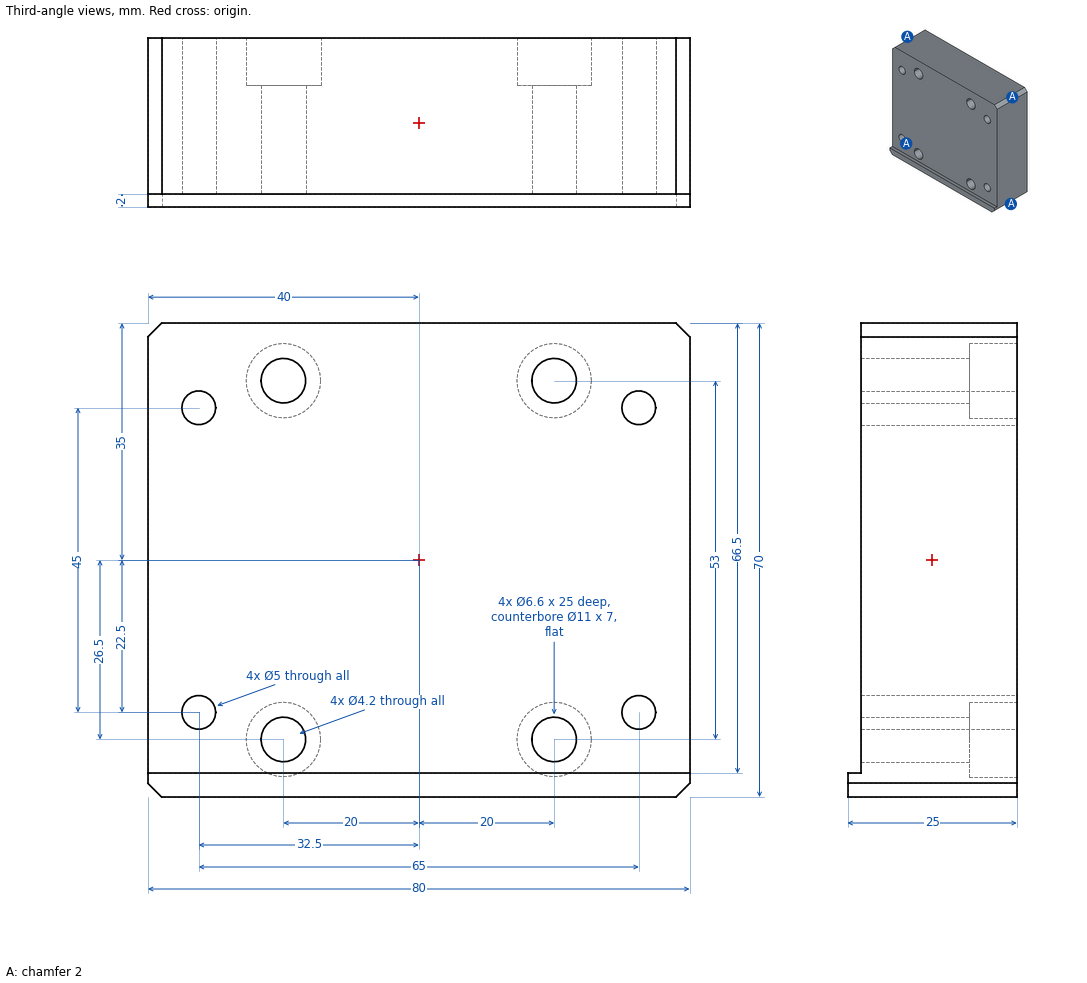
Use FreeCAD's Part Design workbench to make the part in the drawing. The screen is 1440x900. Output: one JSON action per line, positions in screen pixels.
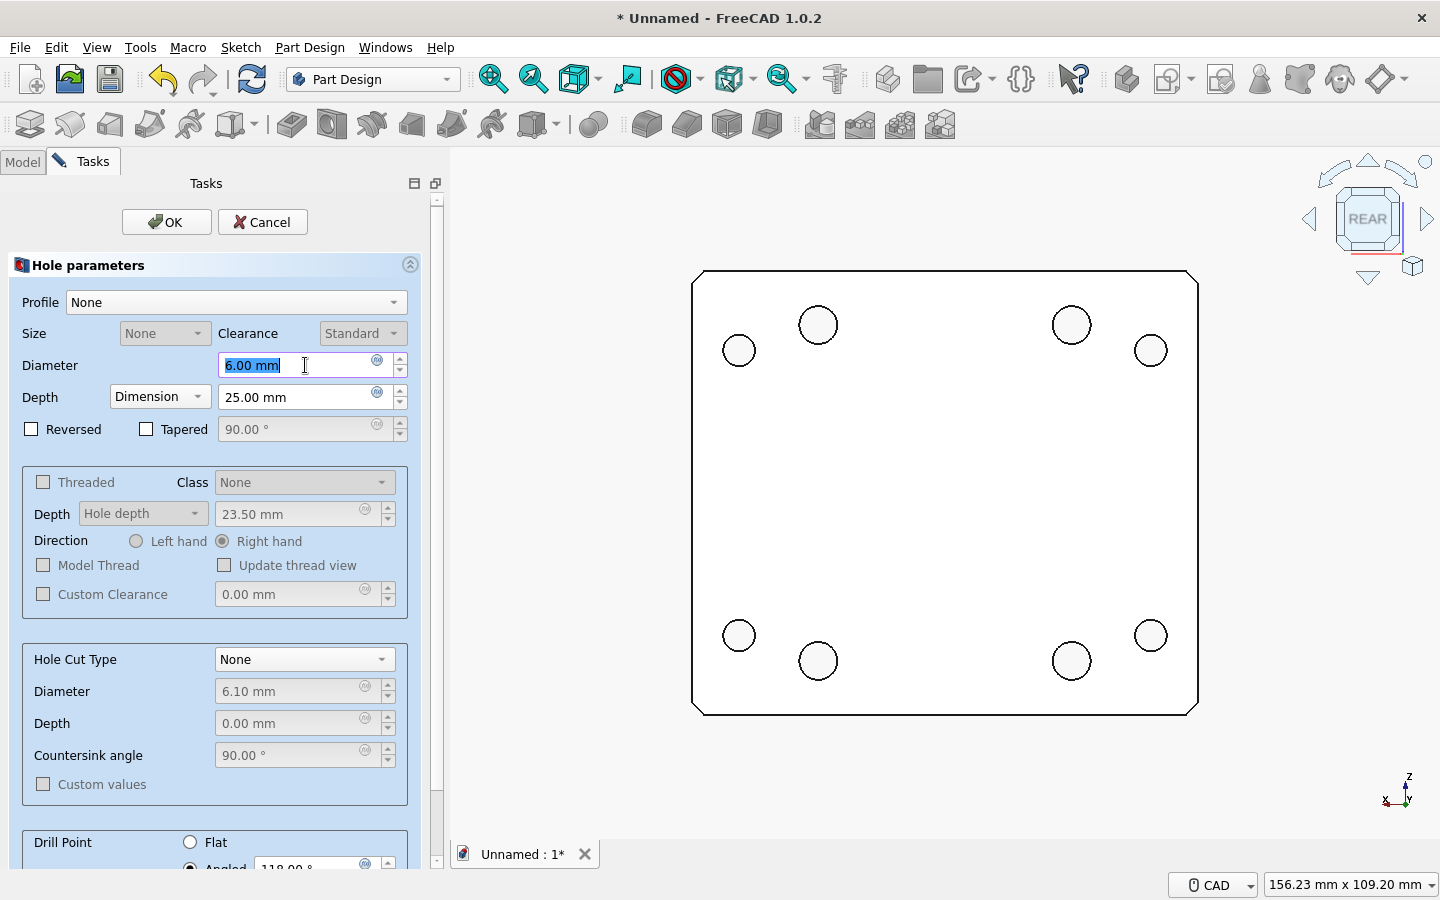
{"action": "type", "text": "6.6"}
{"action": "key", "text": "Tab"}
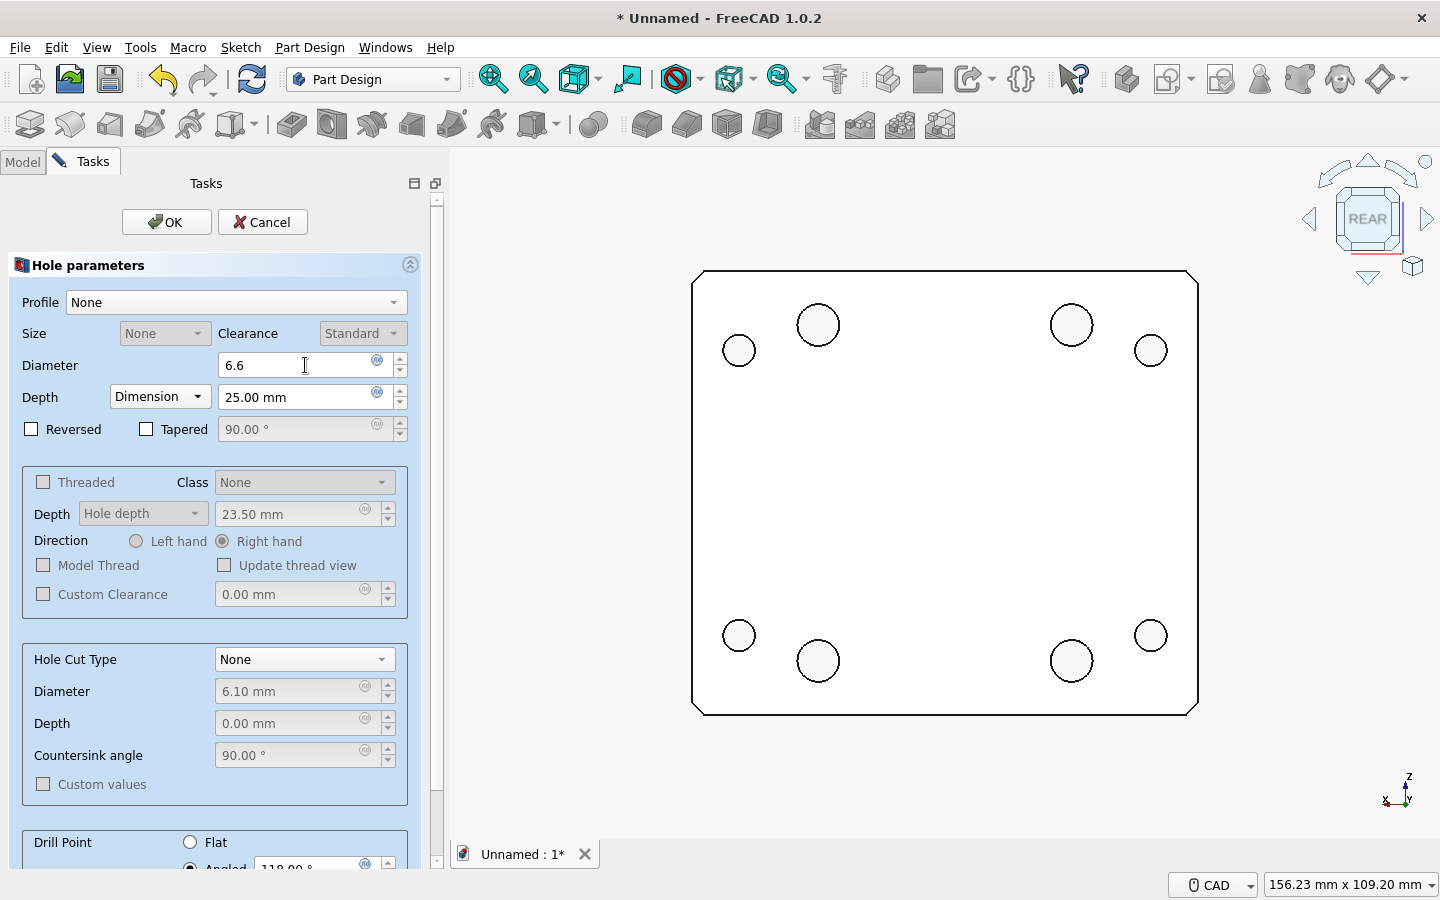
{"action": "triple_click", "coordinate": [305, 397]}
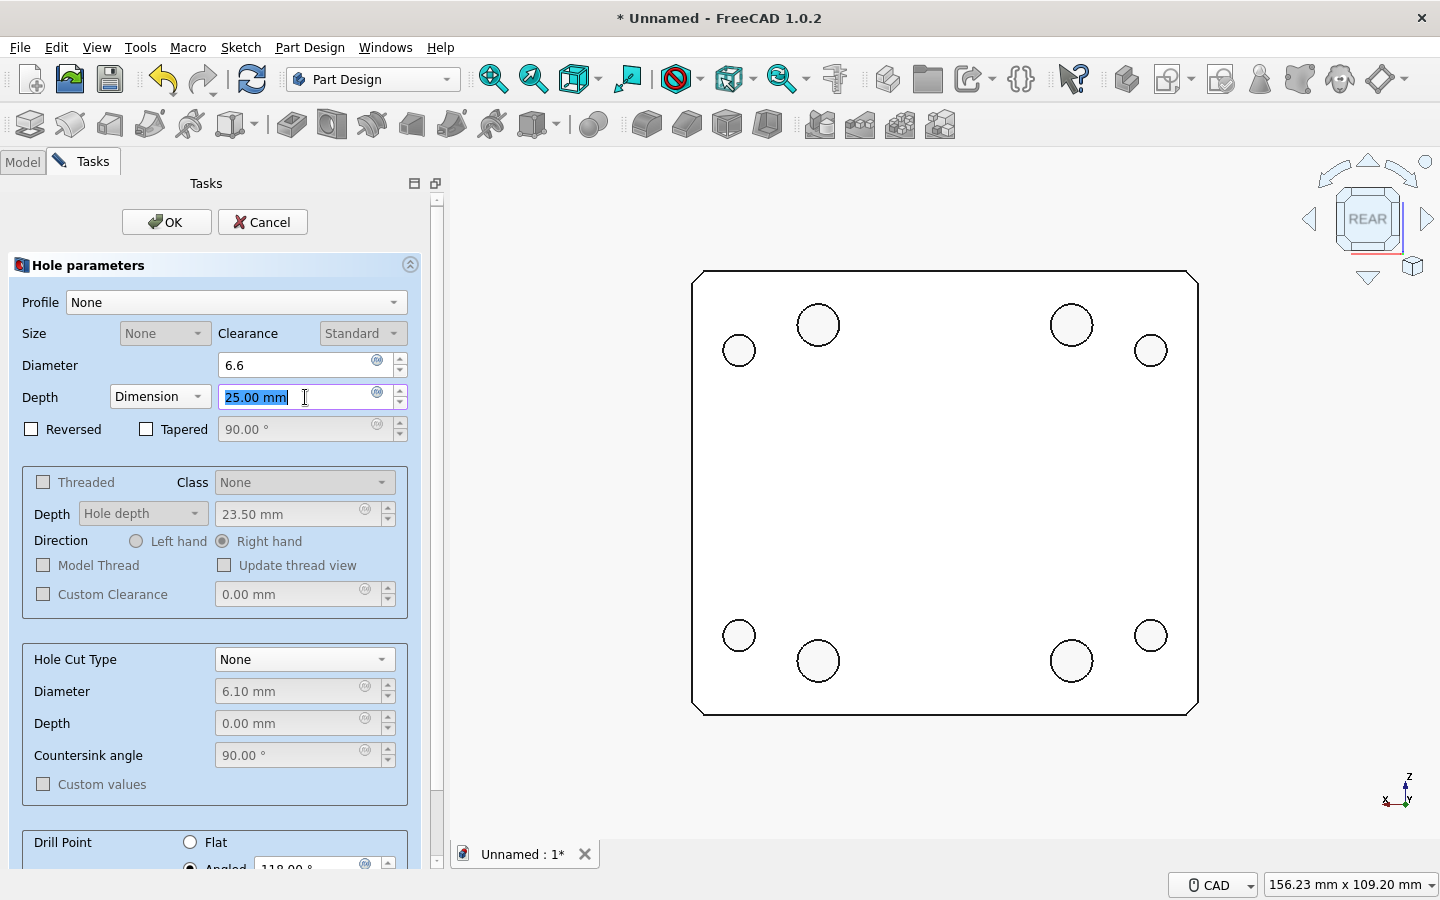
{"action": "type", "text": "25"}
{"action": "key", "text": "Tab"}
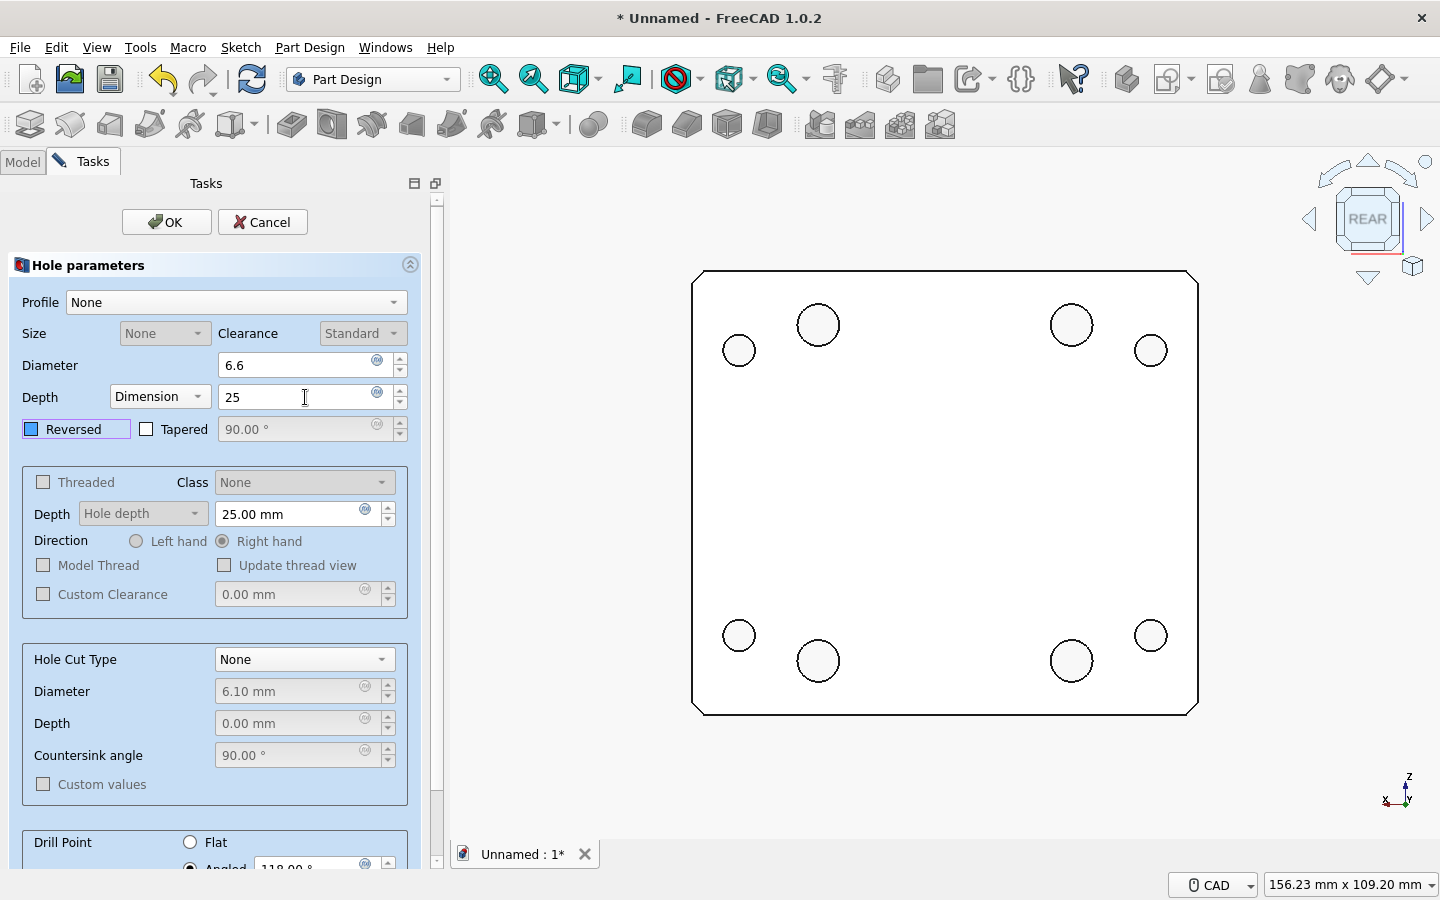
{"action": "left_click", "coordinate": [306, 660]}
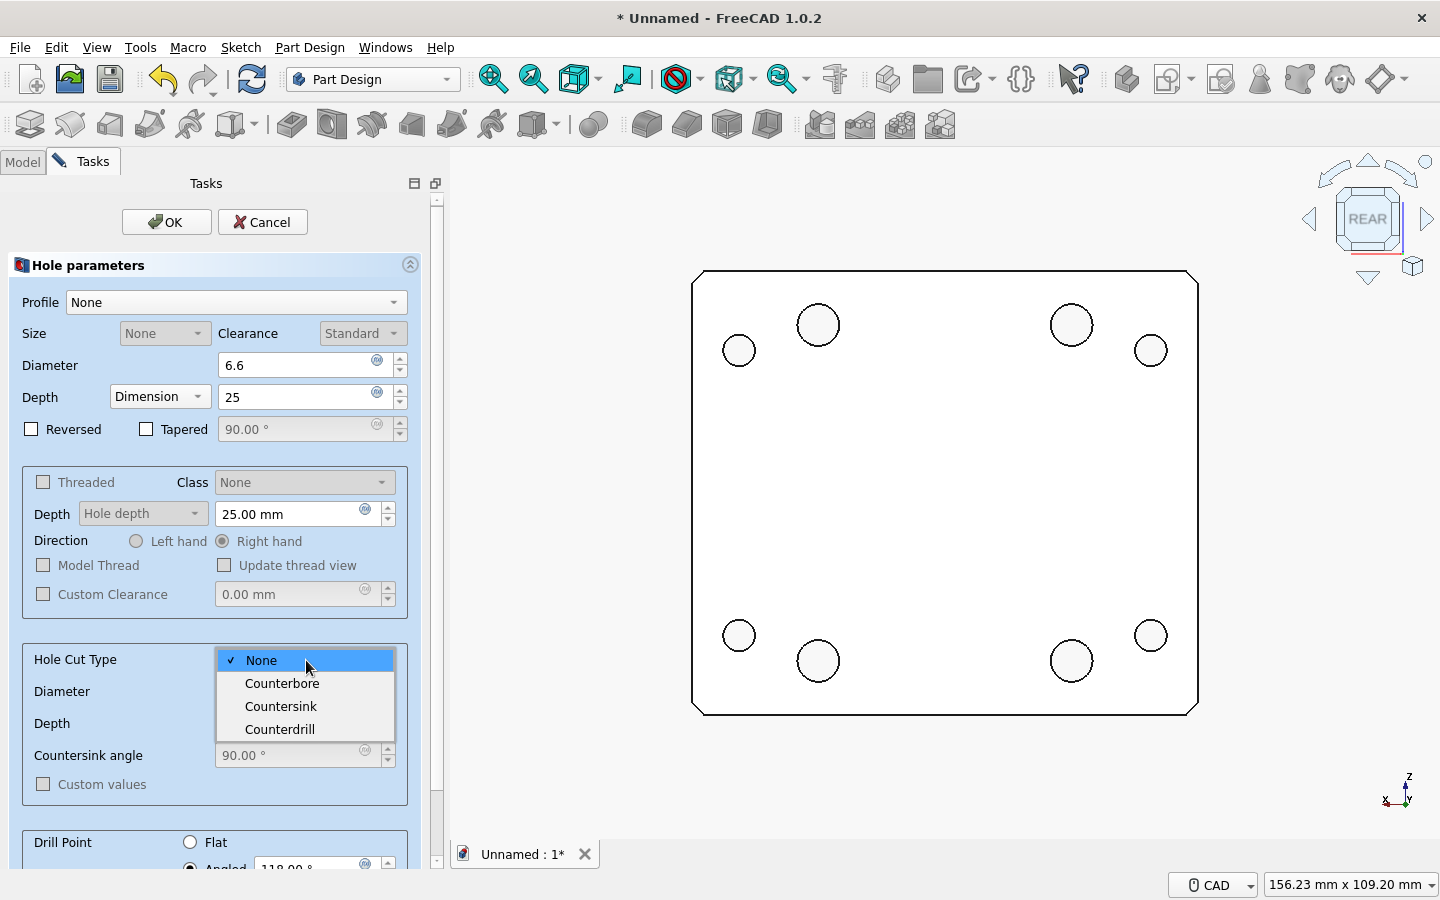
{"action": "left_click", "coordinate": [304, 684]}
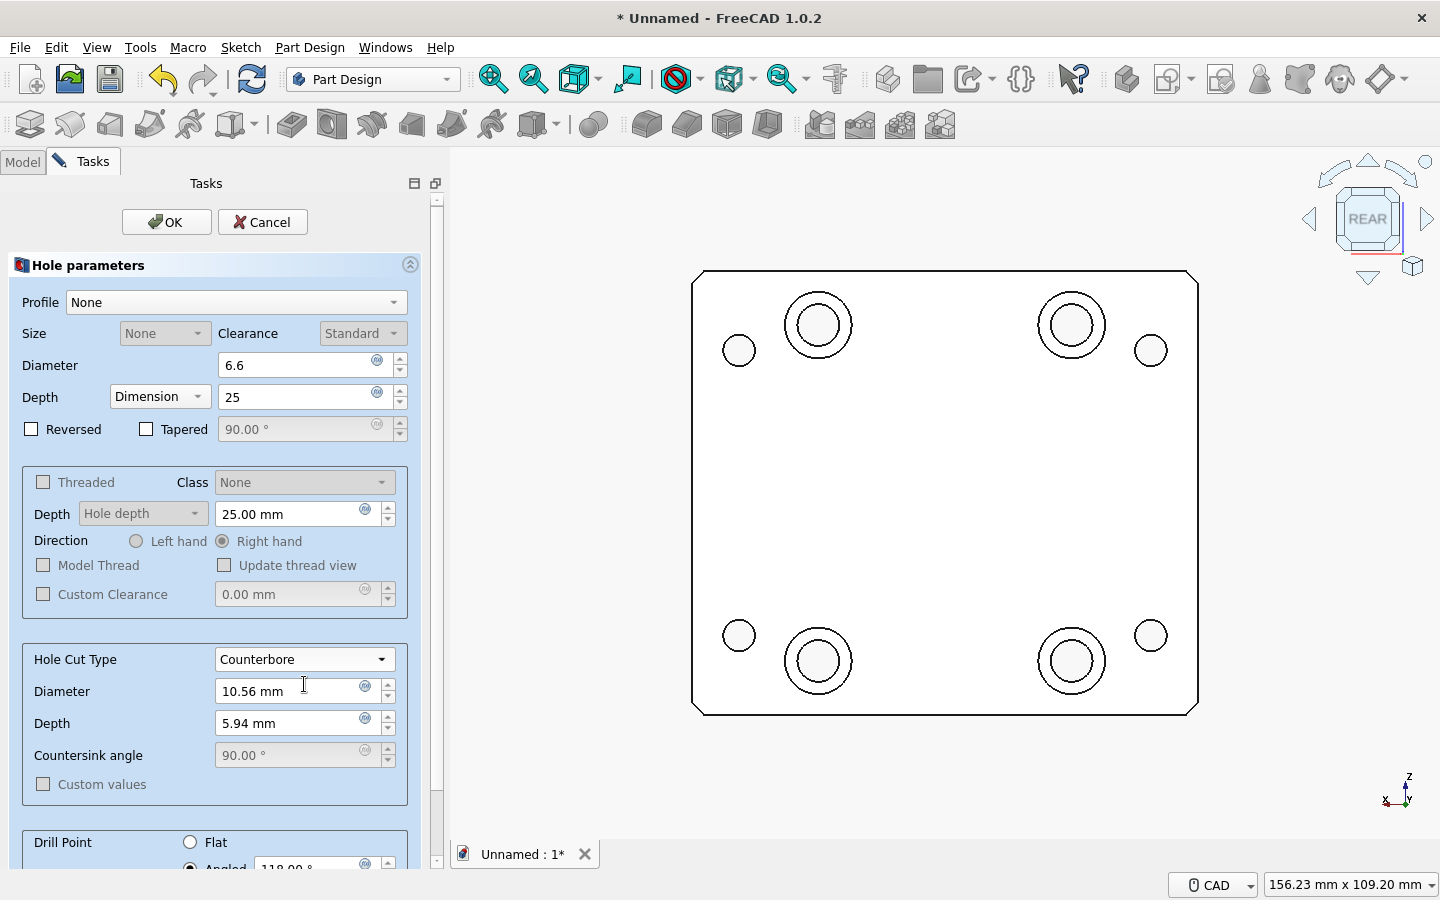
{"action": "triple_click", "coordinate": [298, 691]}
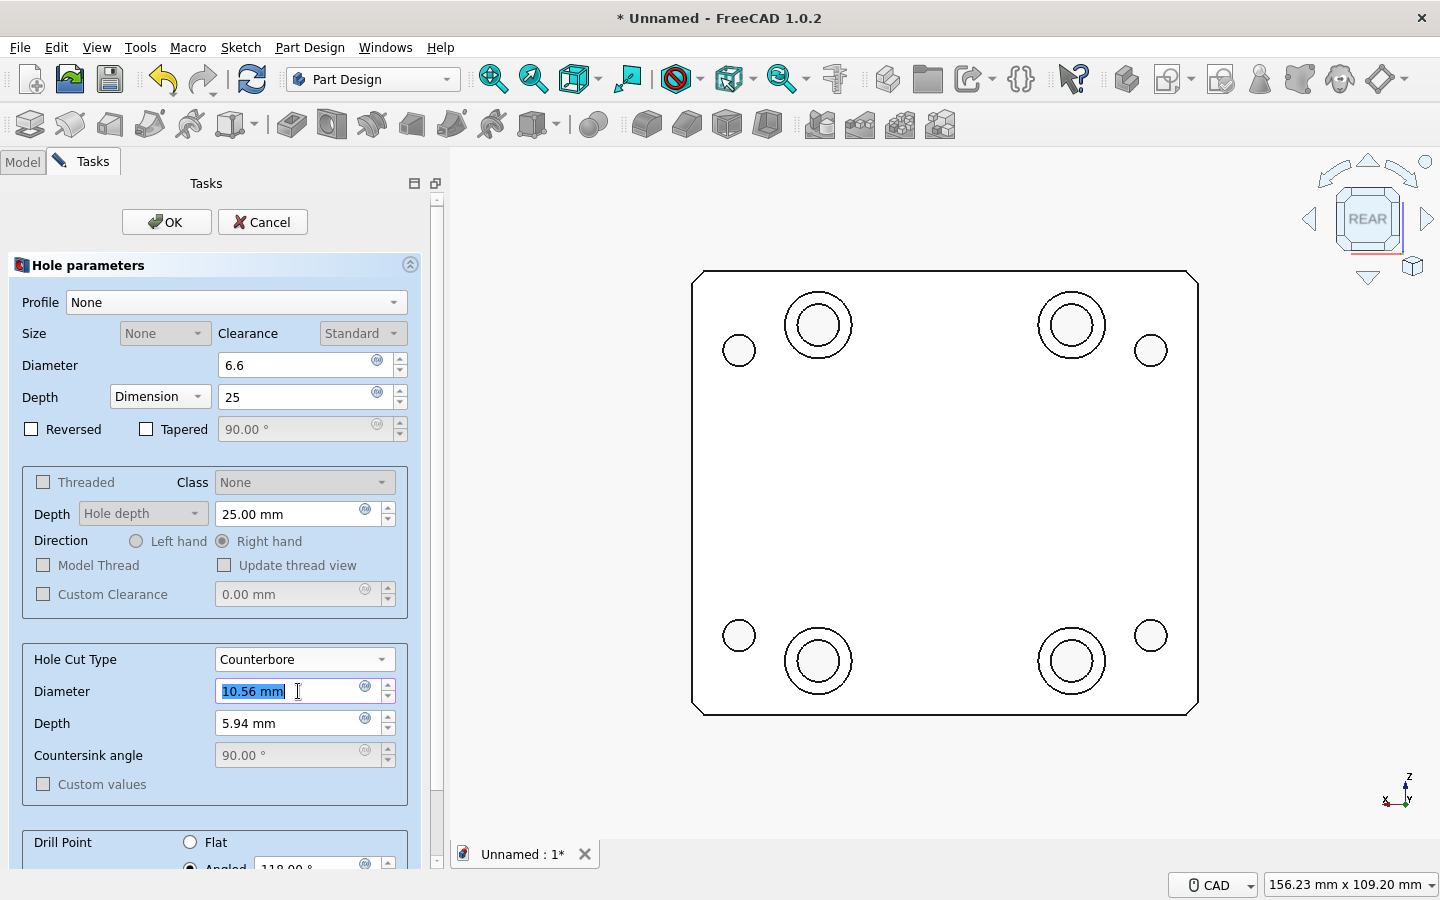
{"action": "type", "text": "11"}
{"action": "key", "text": "Tab"}